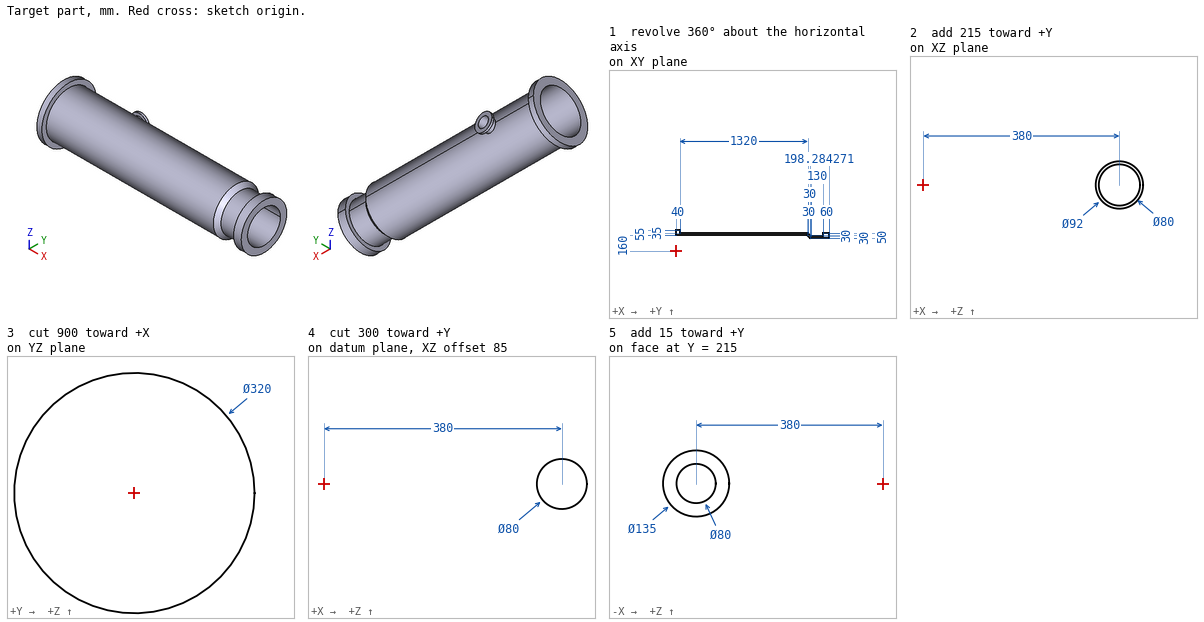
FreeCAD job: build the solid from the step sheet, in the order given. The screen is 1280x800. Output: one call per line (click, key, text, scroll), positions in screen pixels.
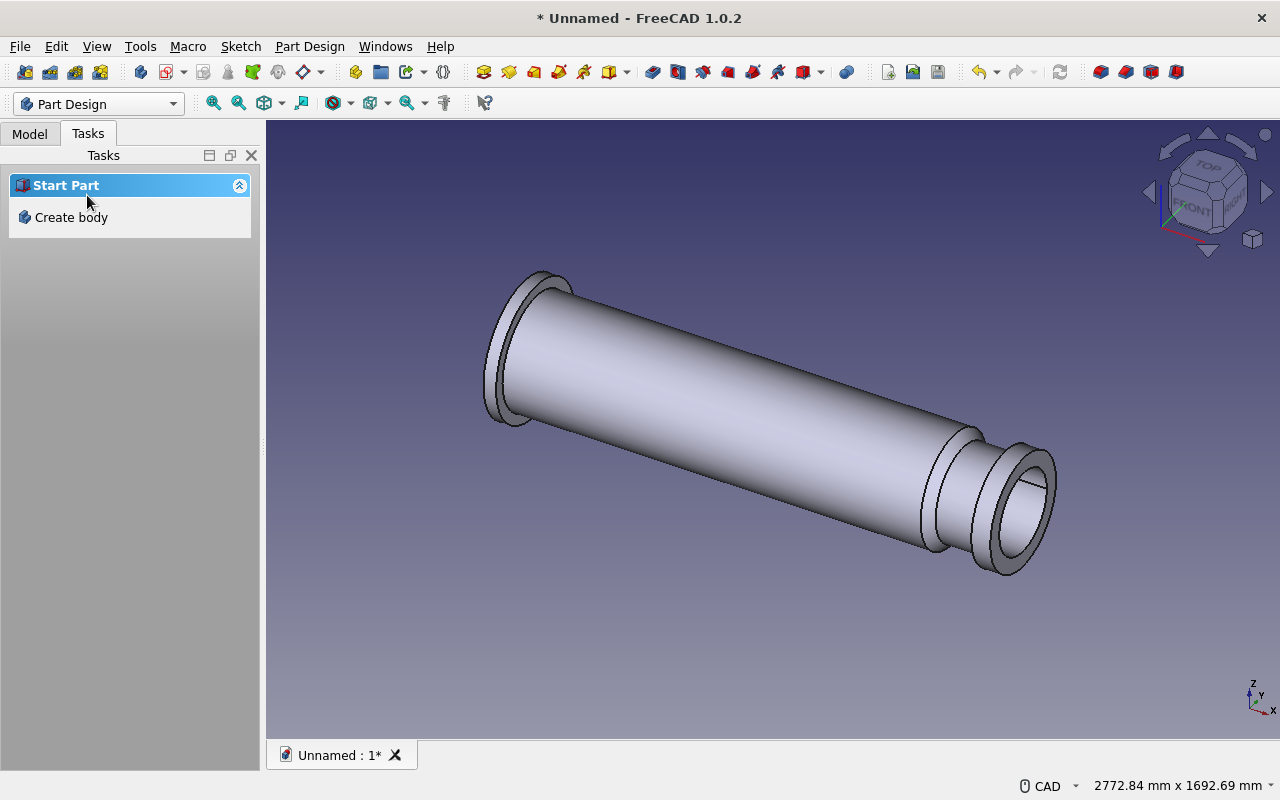
click(166, 72)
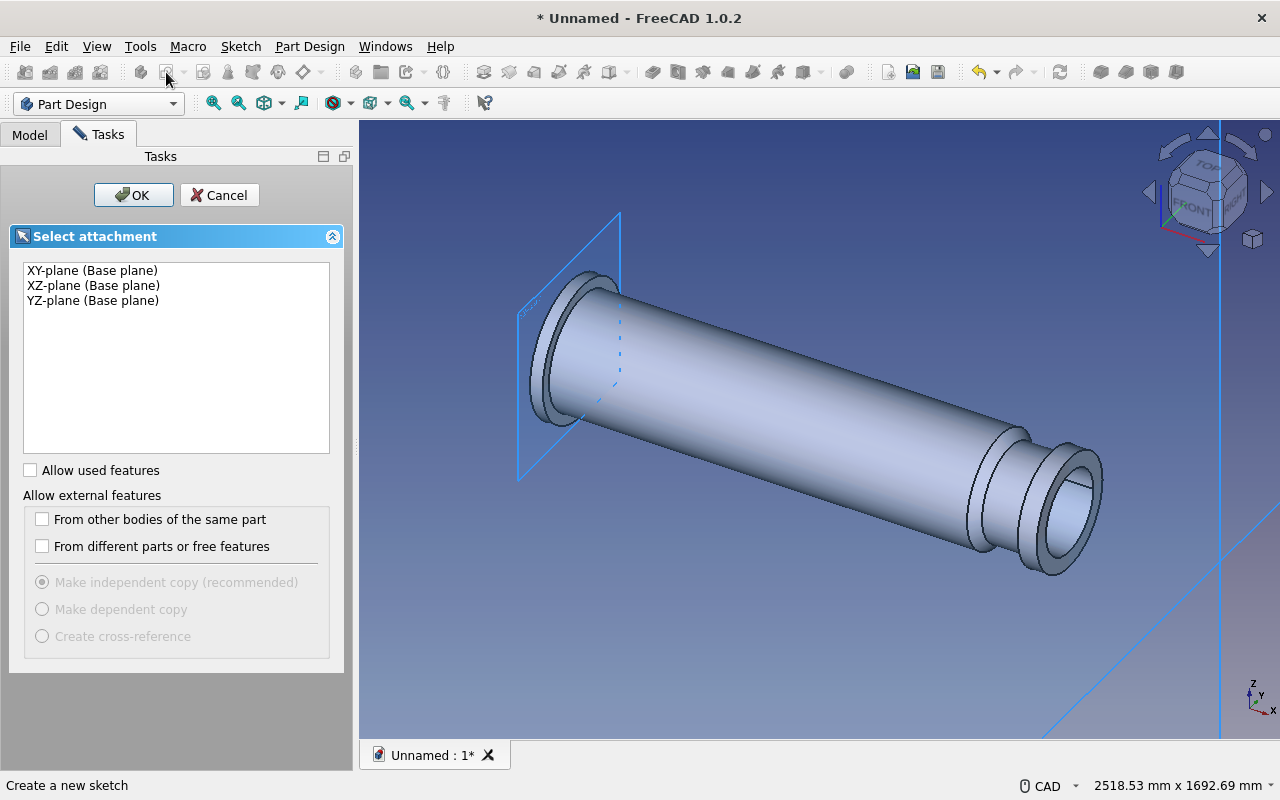
click(84, 286)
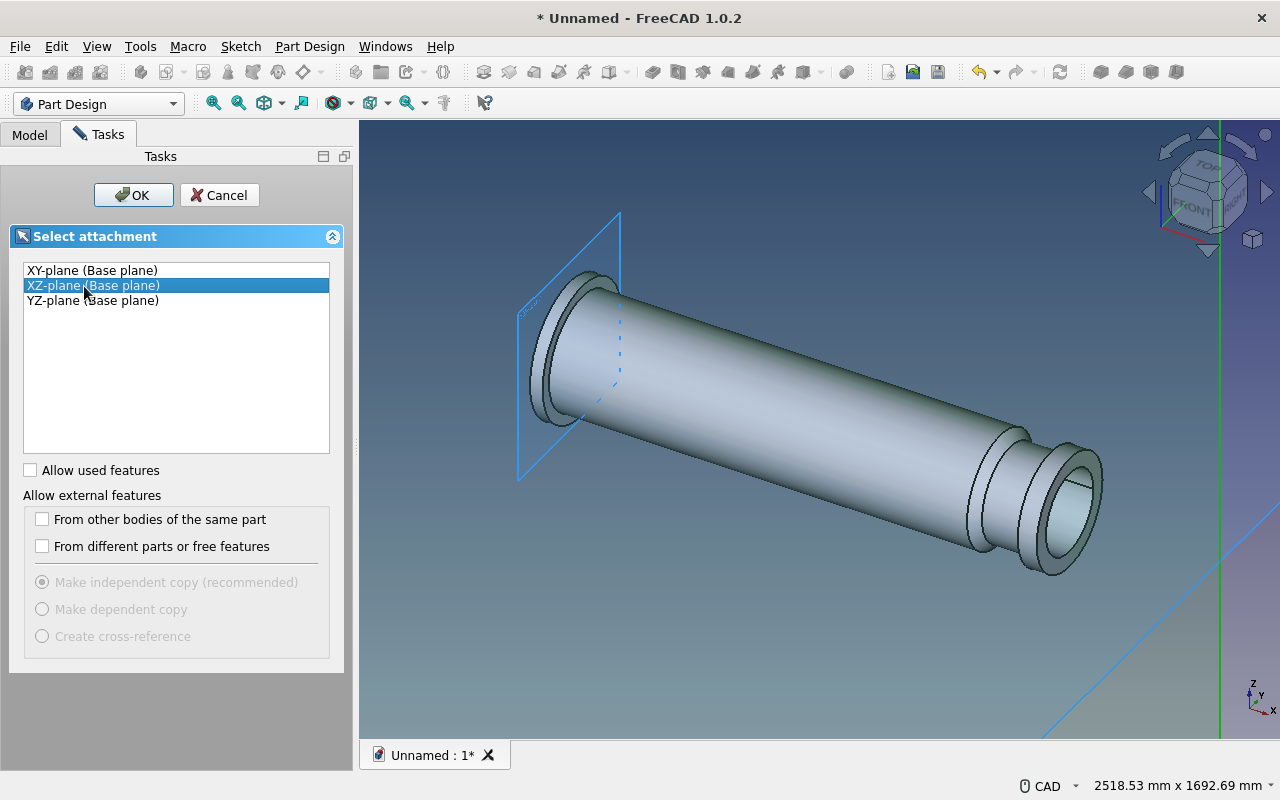
click(134, 195)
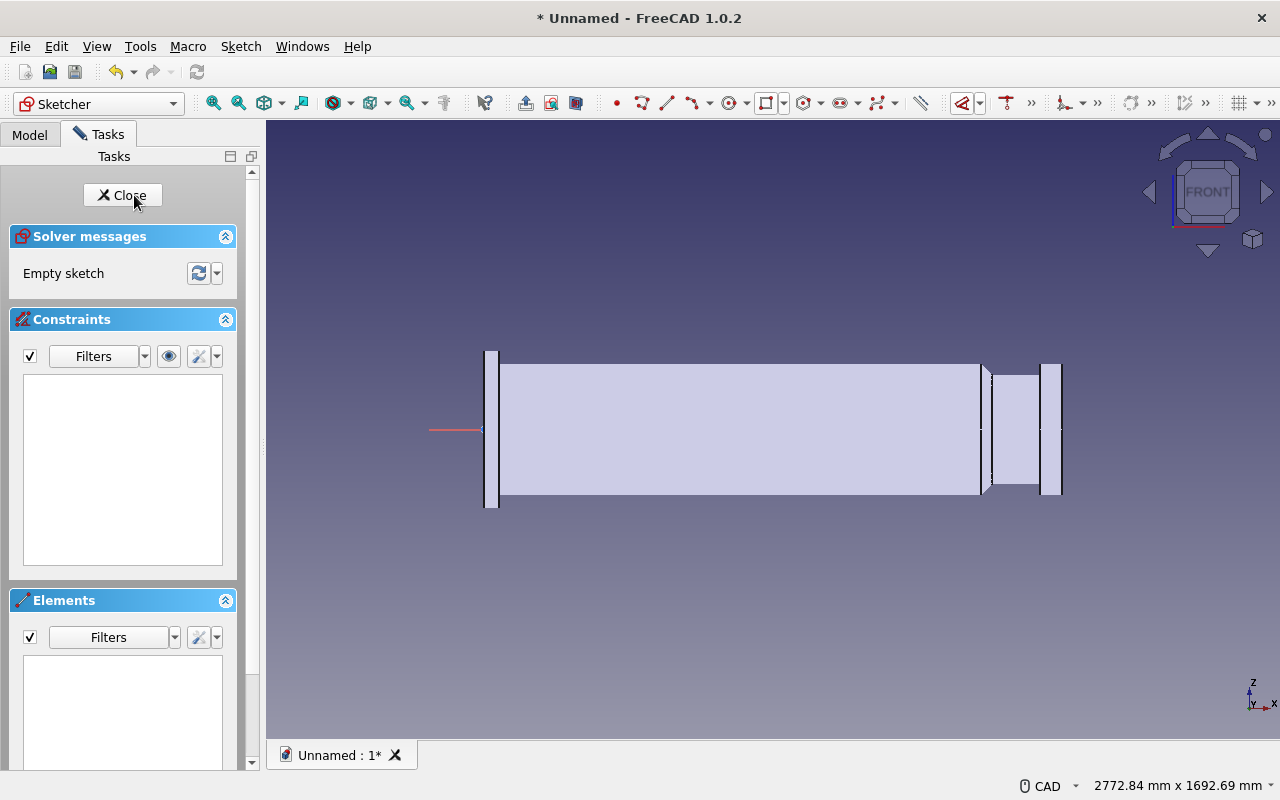
key(q)
key(s)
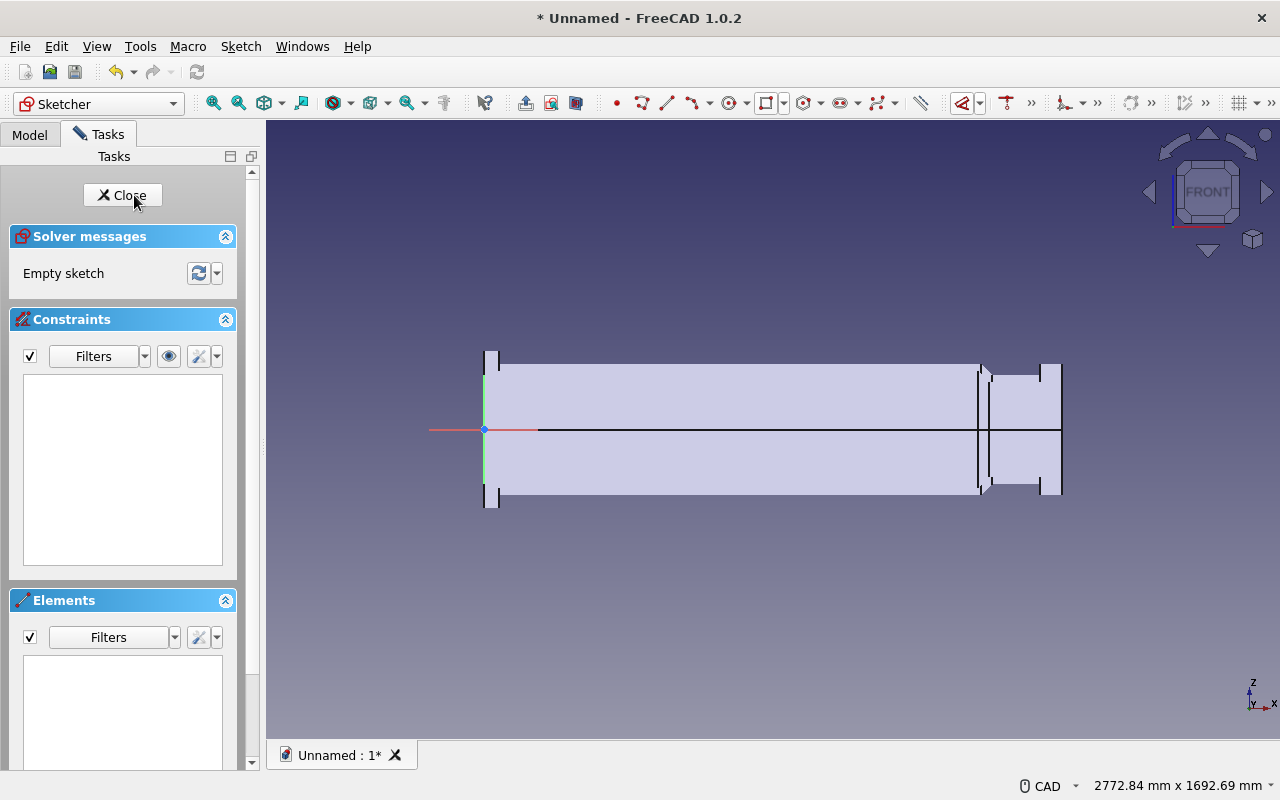
scroll(615, 429, up, 12)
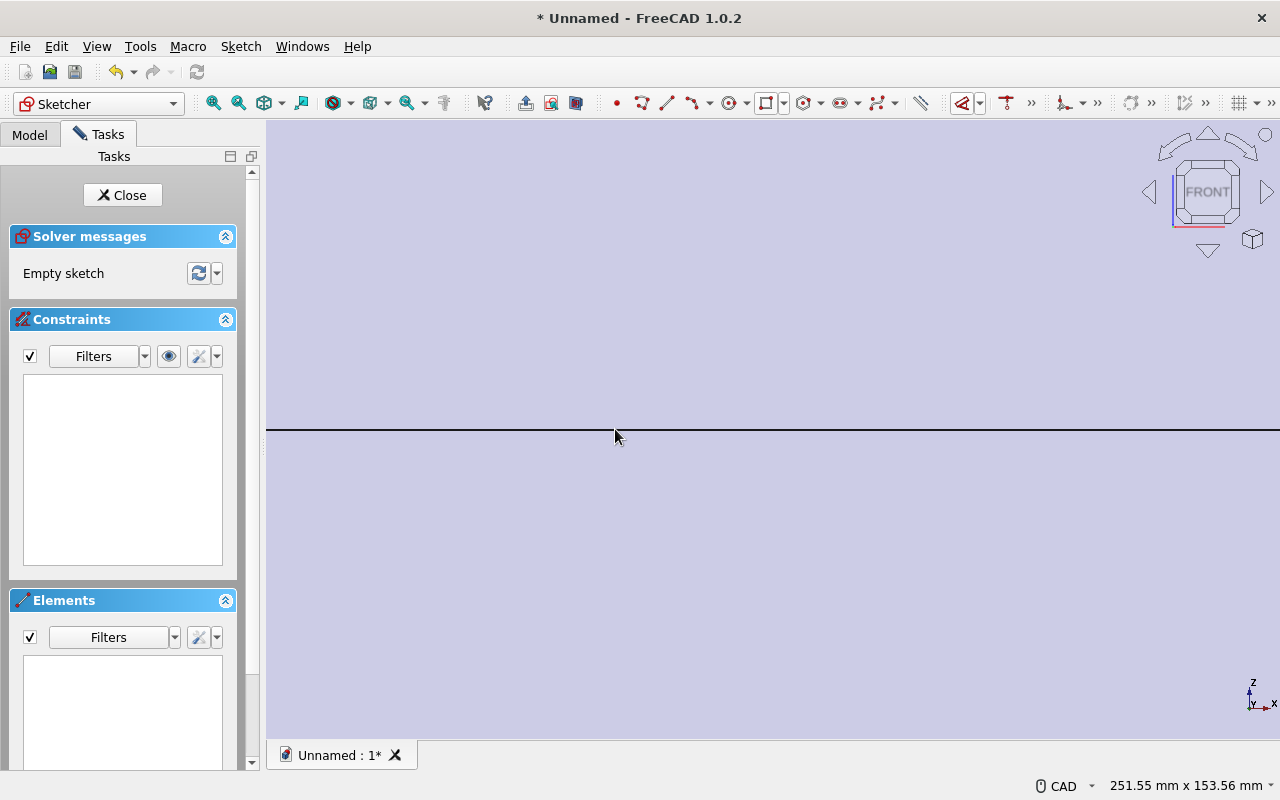
key(g)
key(c)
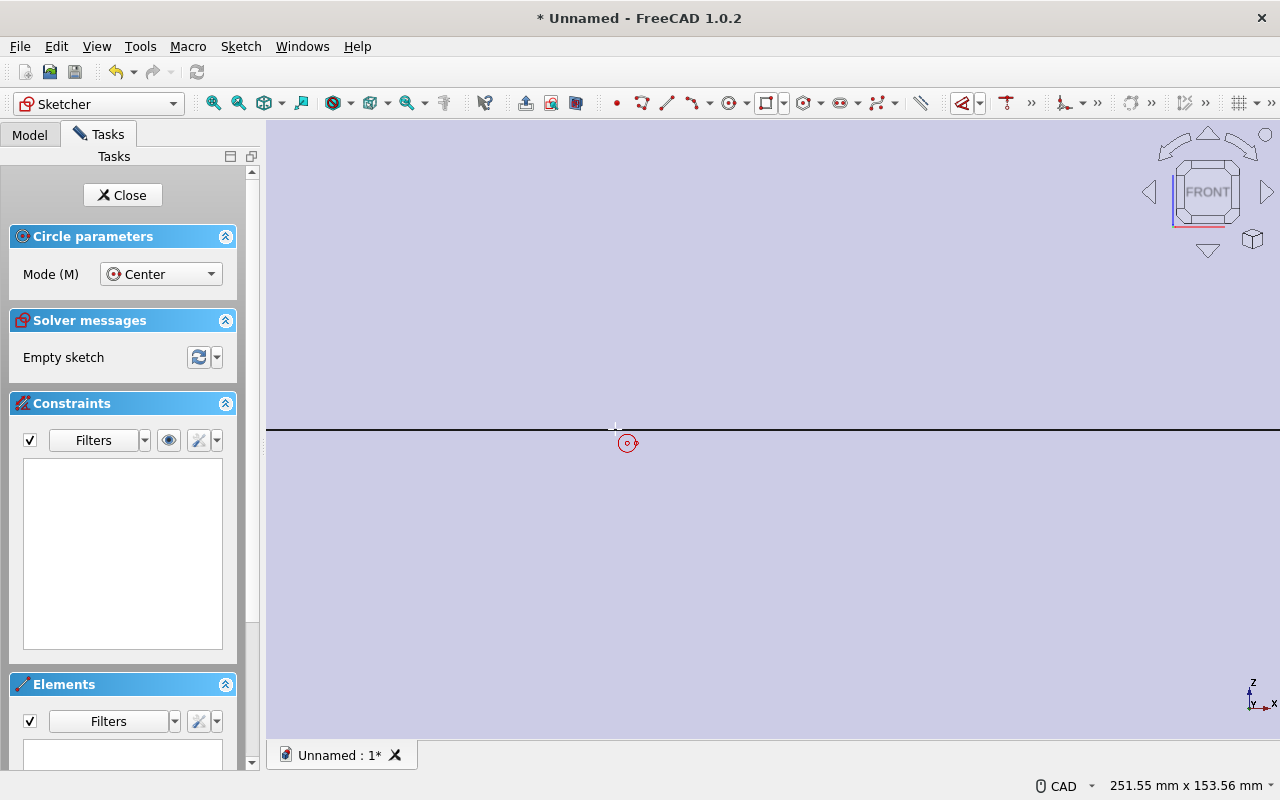
click(700, 430)
move(832, 298)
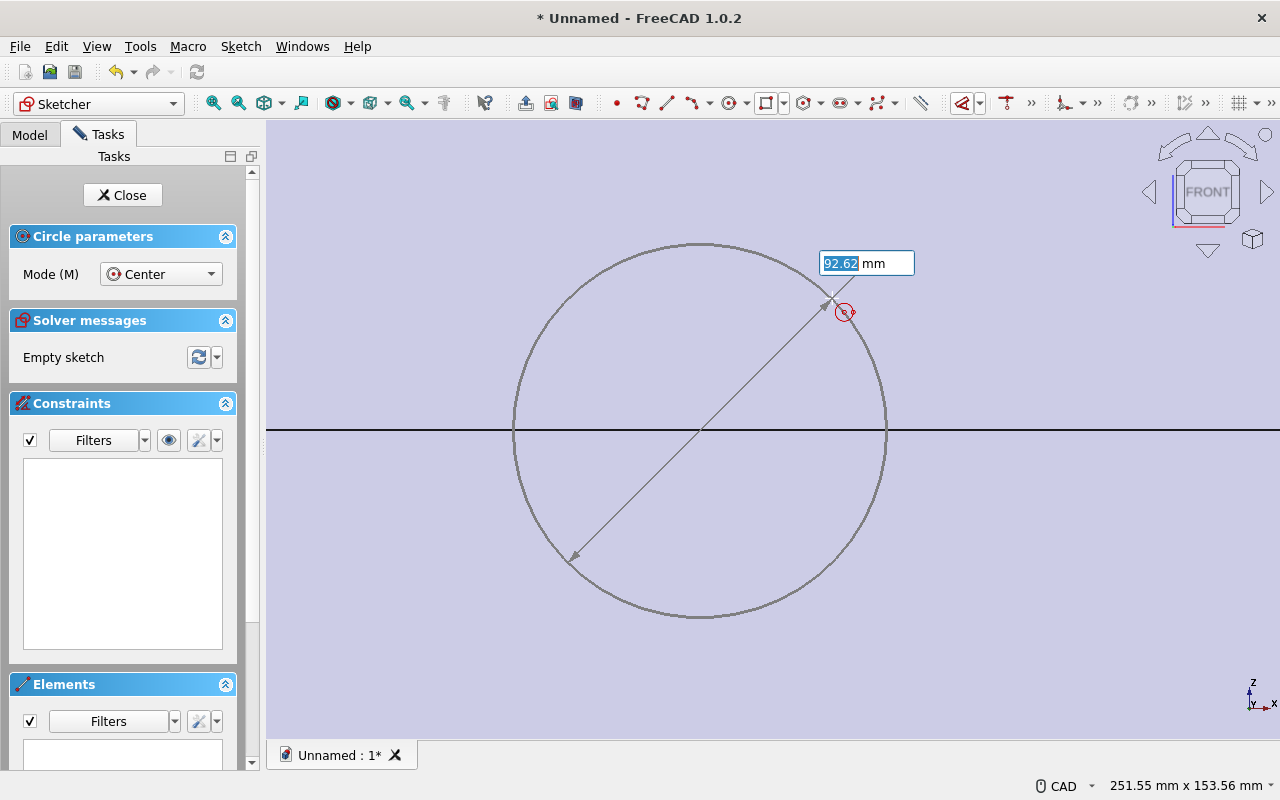
text(92)
key(Return)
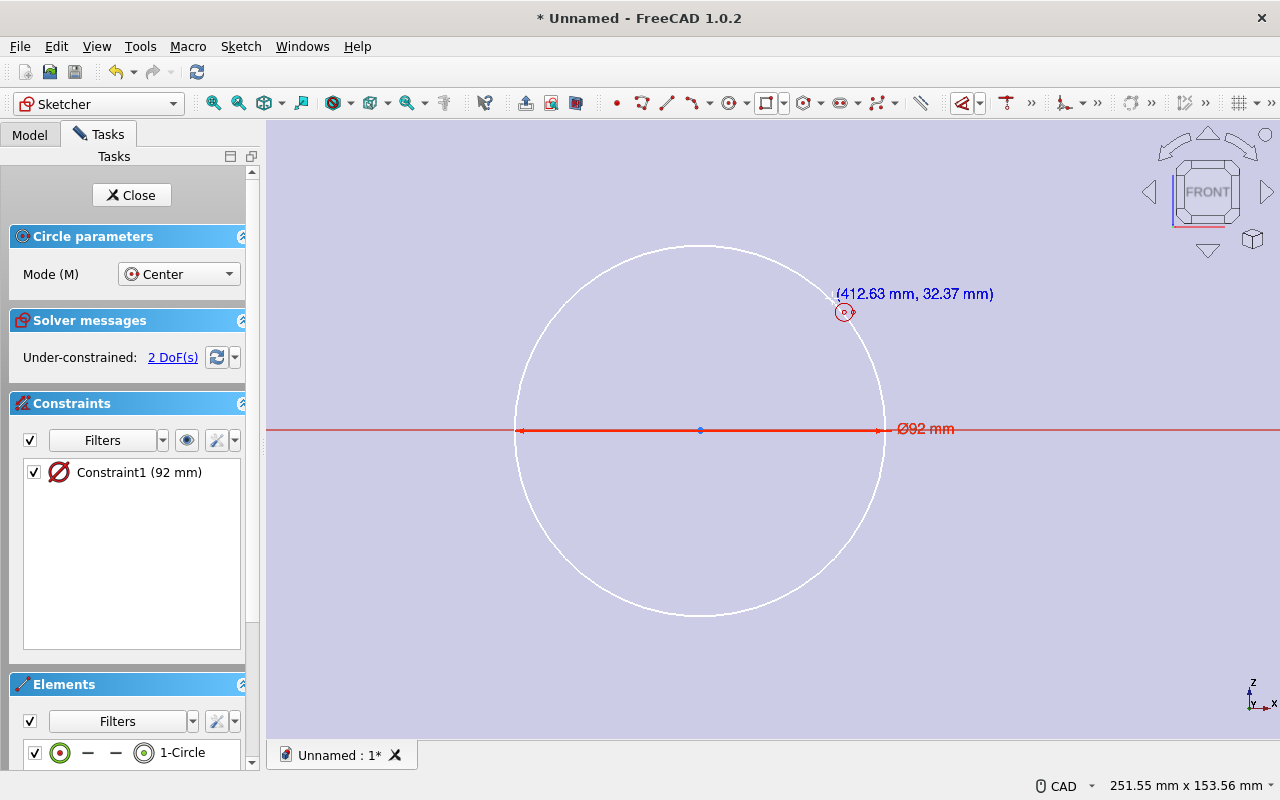
click(700, 431)
move(814, 315)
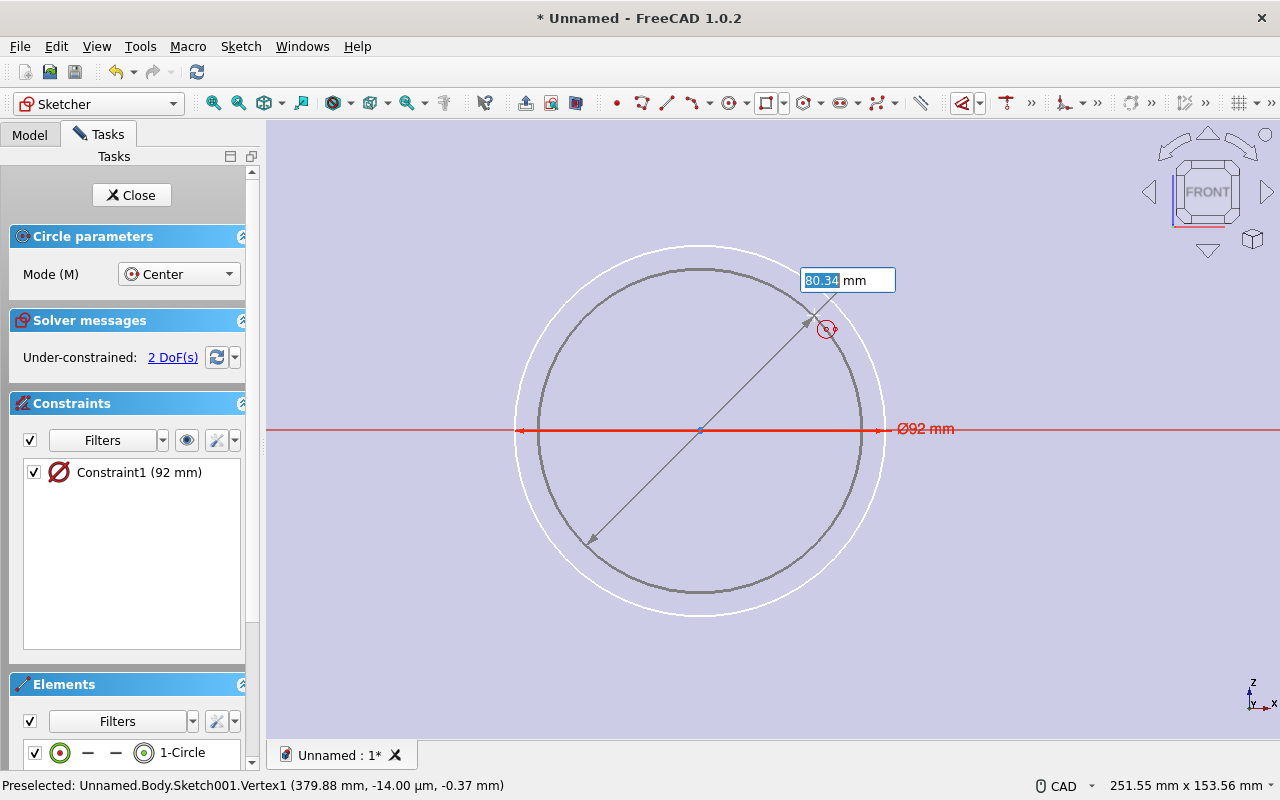
text(80)
key(Return)
key(Escape)